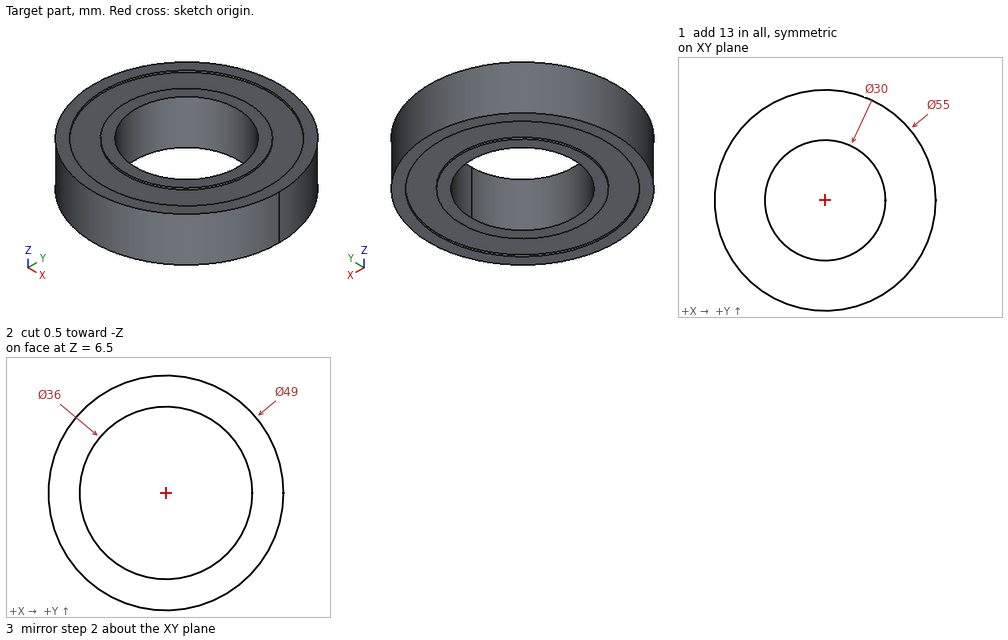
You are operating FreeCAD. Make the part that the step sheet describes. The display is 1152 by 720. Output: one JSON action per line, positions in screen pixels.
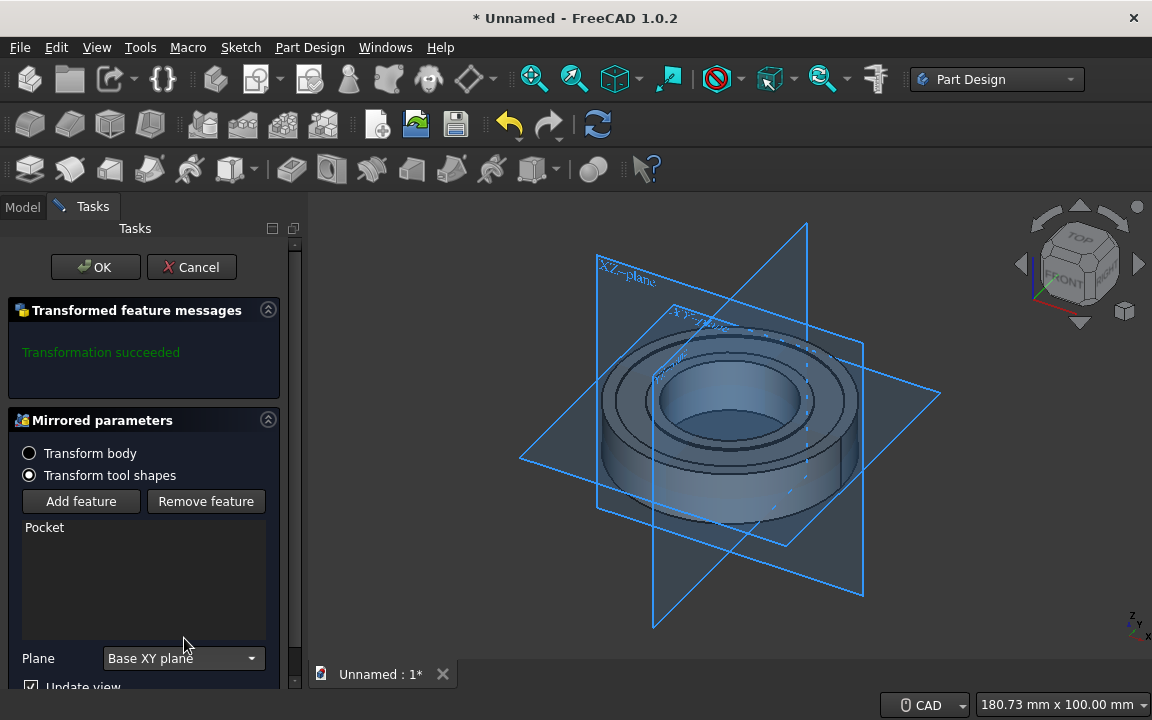
{"action": "left_click", "coordinate": [96, 267]}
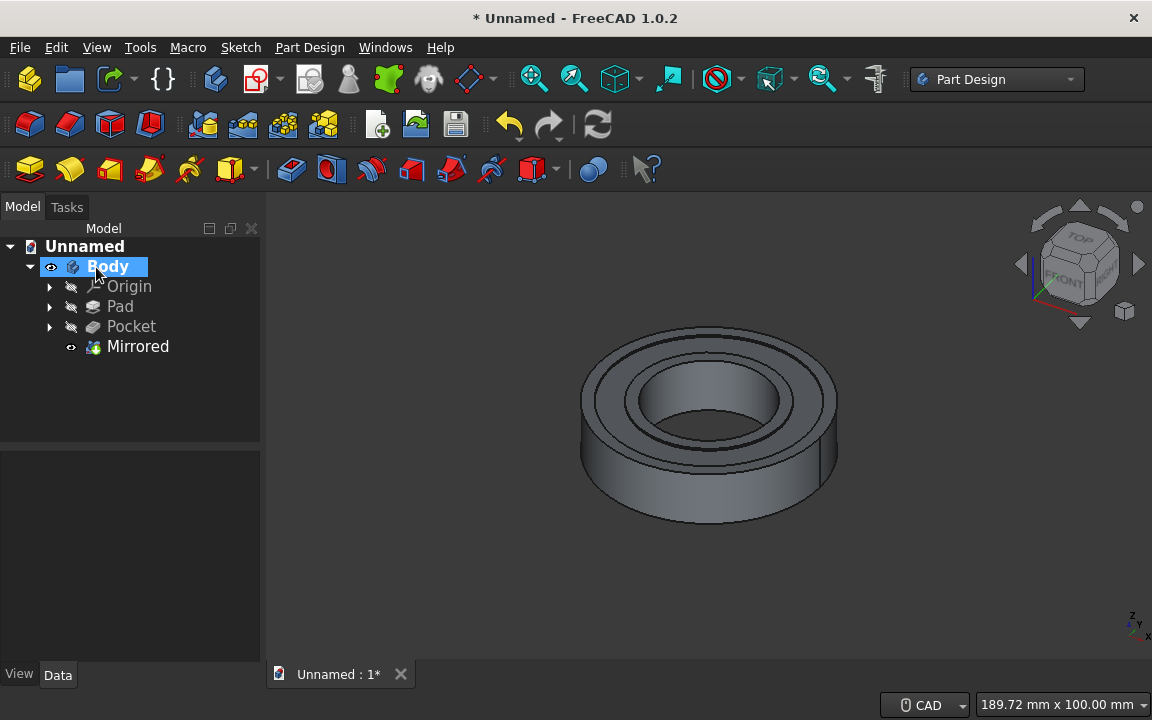
{"action": "key", "text": "0"}